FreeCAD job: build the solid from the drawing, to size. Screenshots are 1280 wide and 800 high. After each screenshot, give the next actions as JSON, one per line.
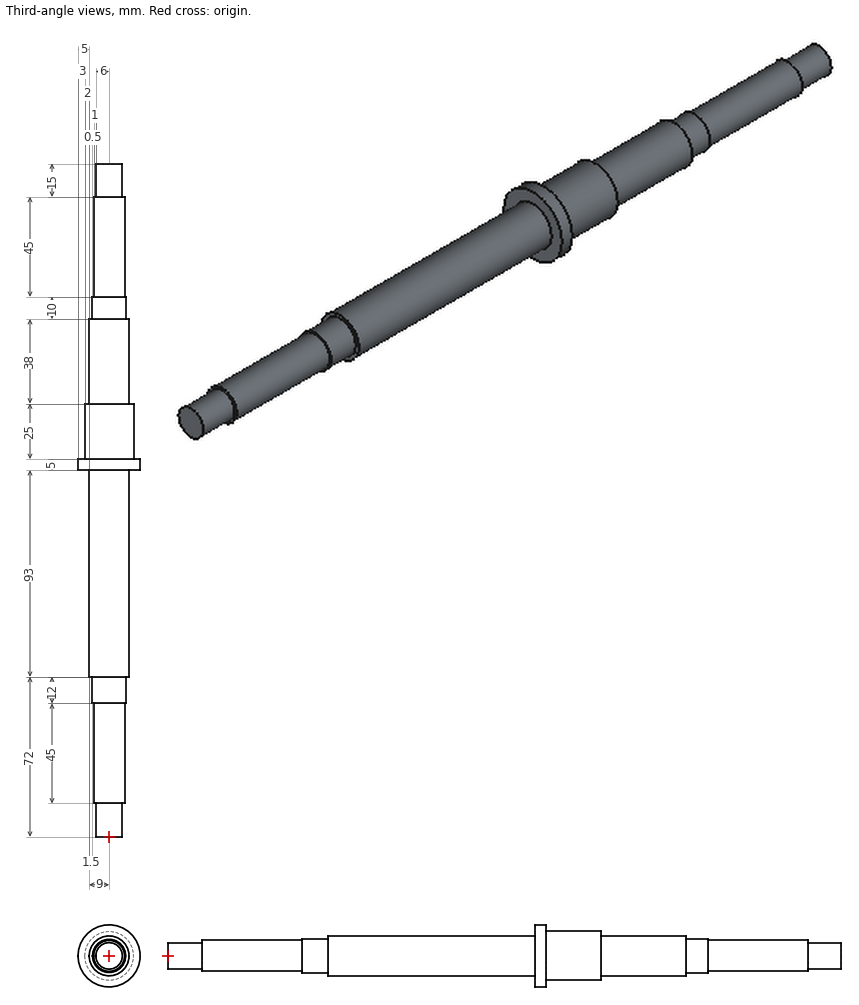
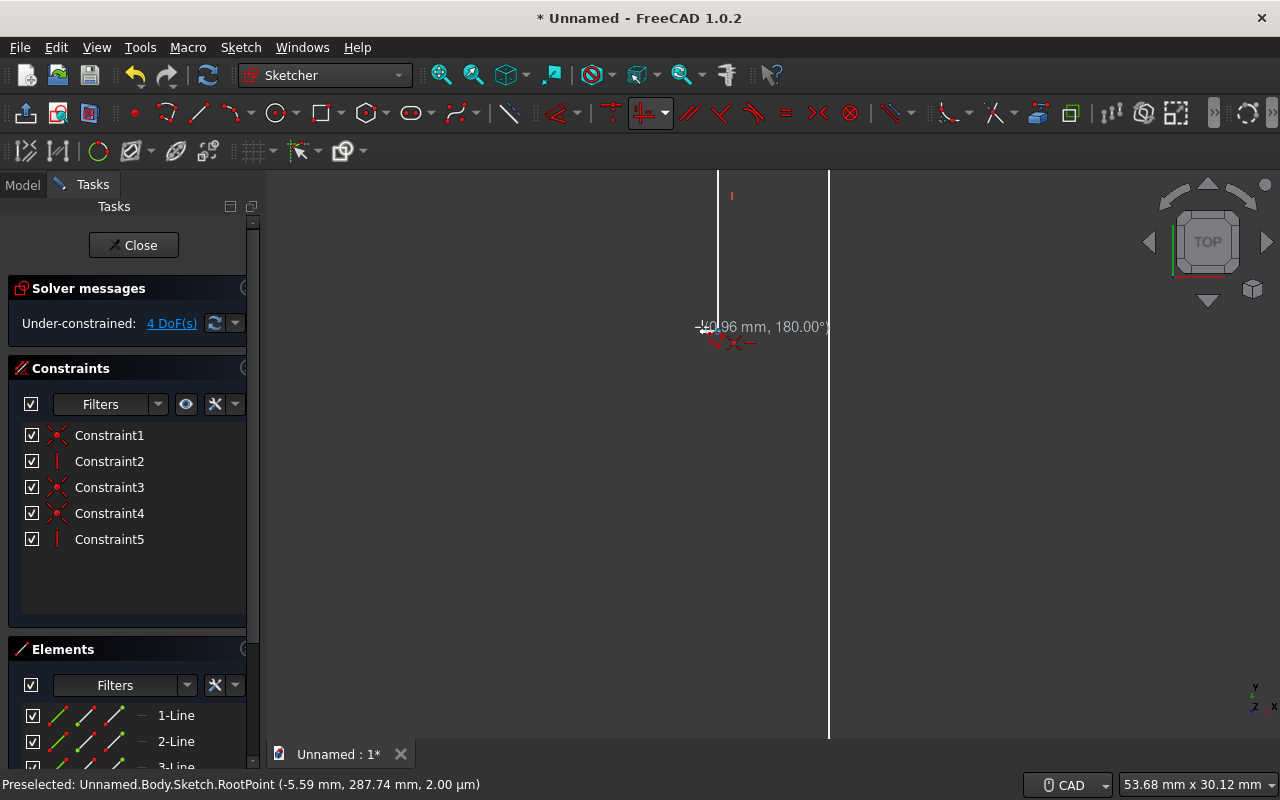
{"action": "left_click", "coordinate": [697, 326]}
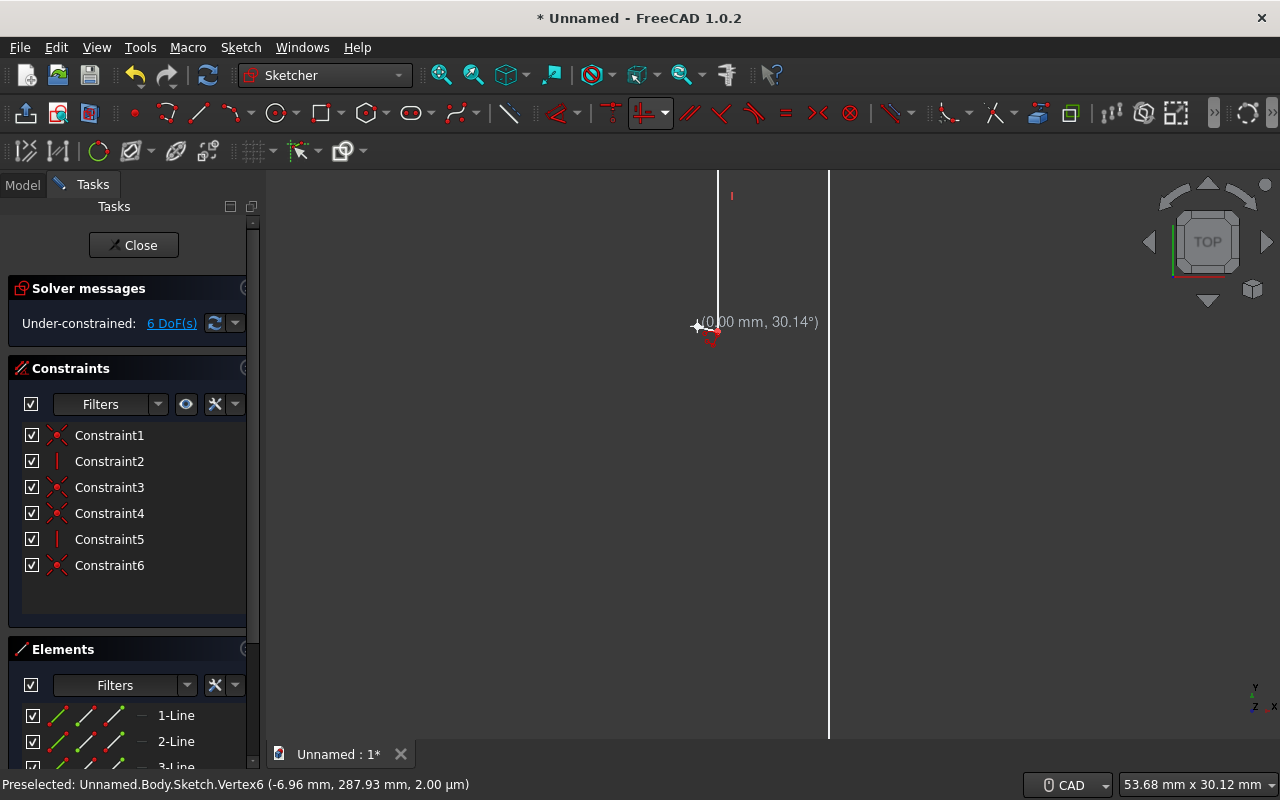
{"action": "scroll", "coordinate": [705, 296], "scroll_direction": "down", "scroll_amount": 14}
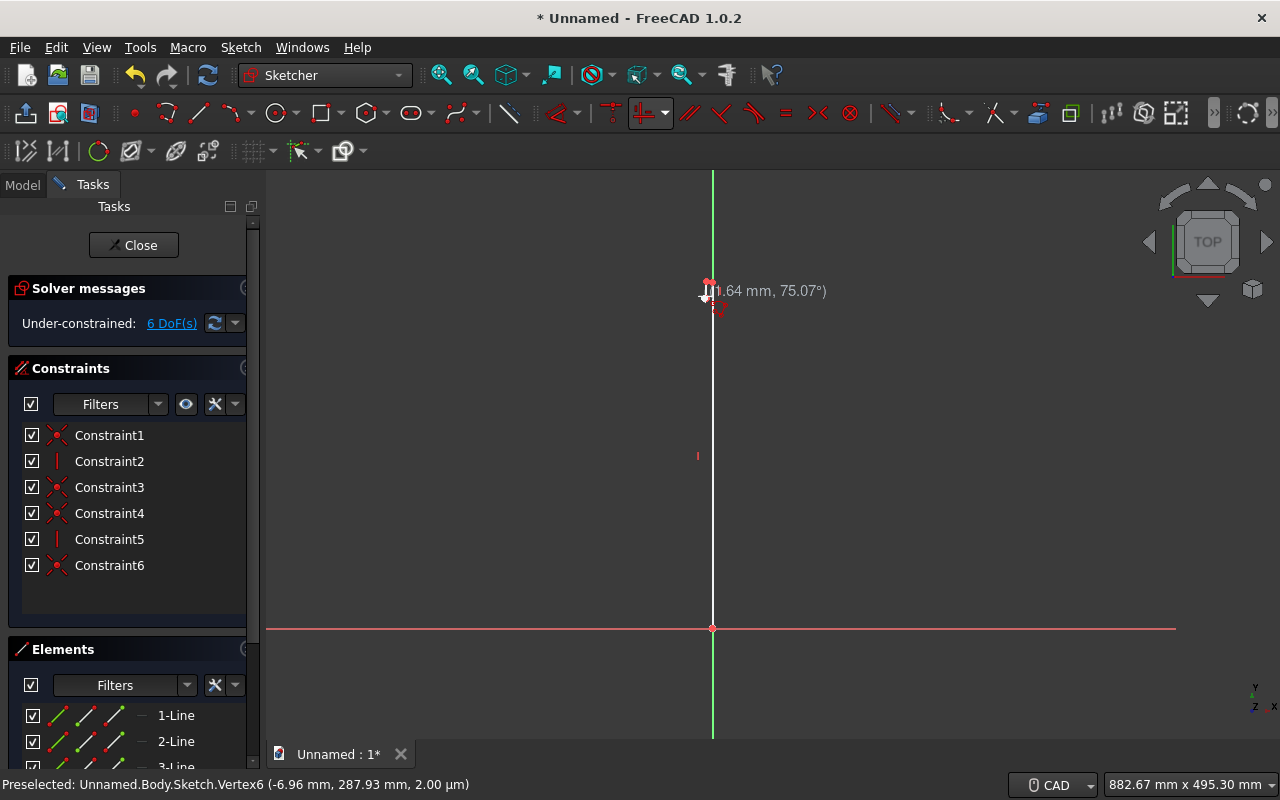
{"action": "scroll", "coordinate": [705, 350], "scroll_direction": "up", "scroll_amount": 4}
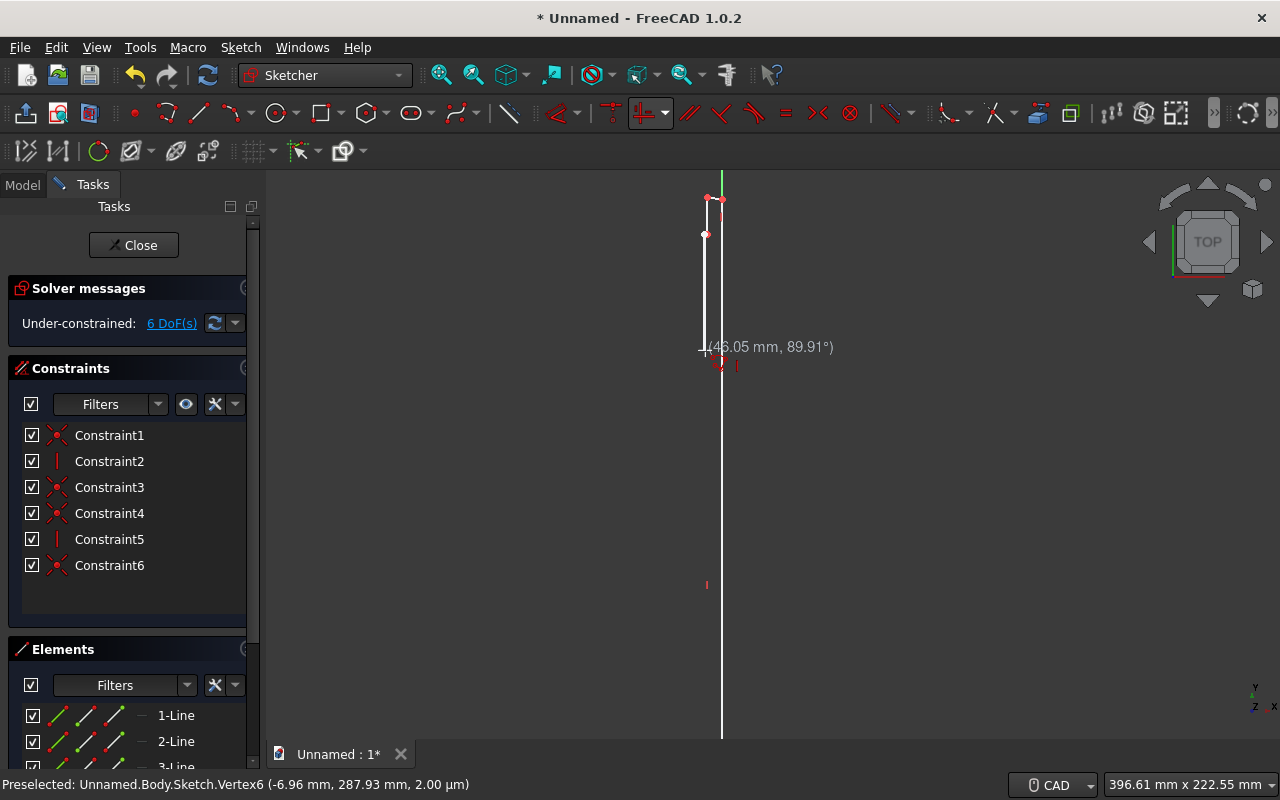
{"action": "left_click", "coordinate": [704, 349]}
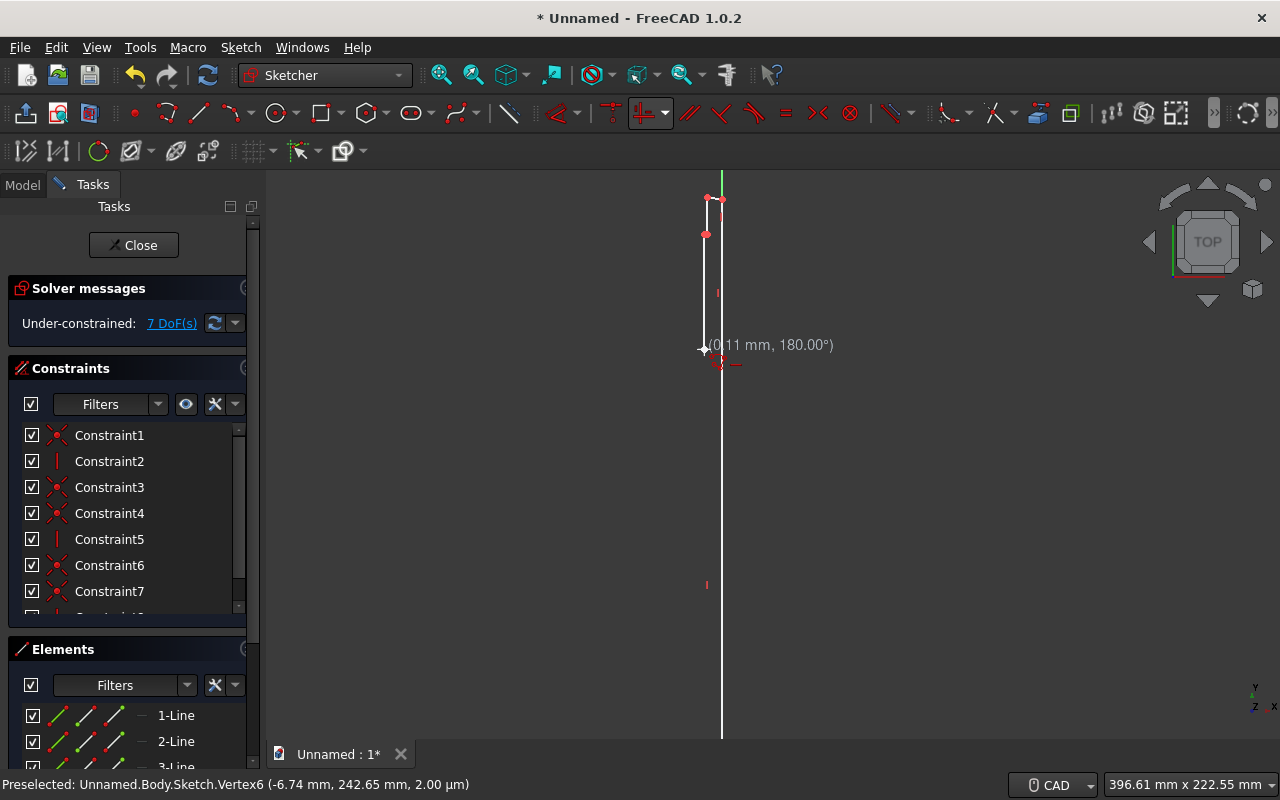
{"action": "scroll", "coordinate": [703, 349], "scroll_direction": "up", "scroll_amount": 13}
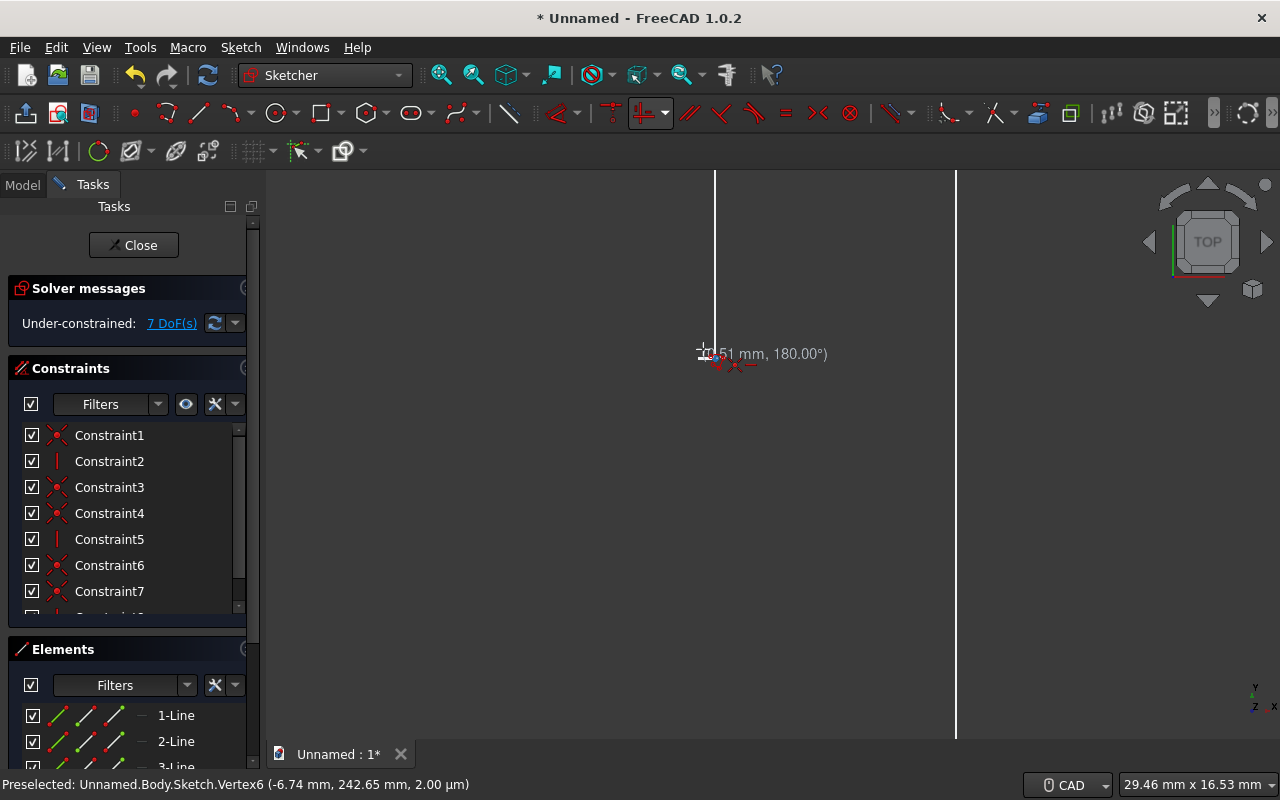
{"action": "left_click", "coordinate": [698, 345]}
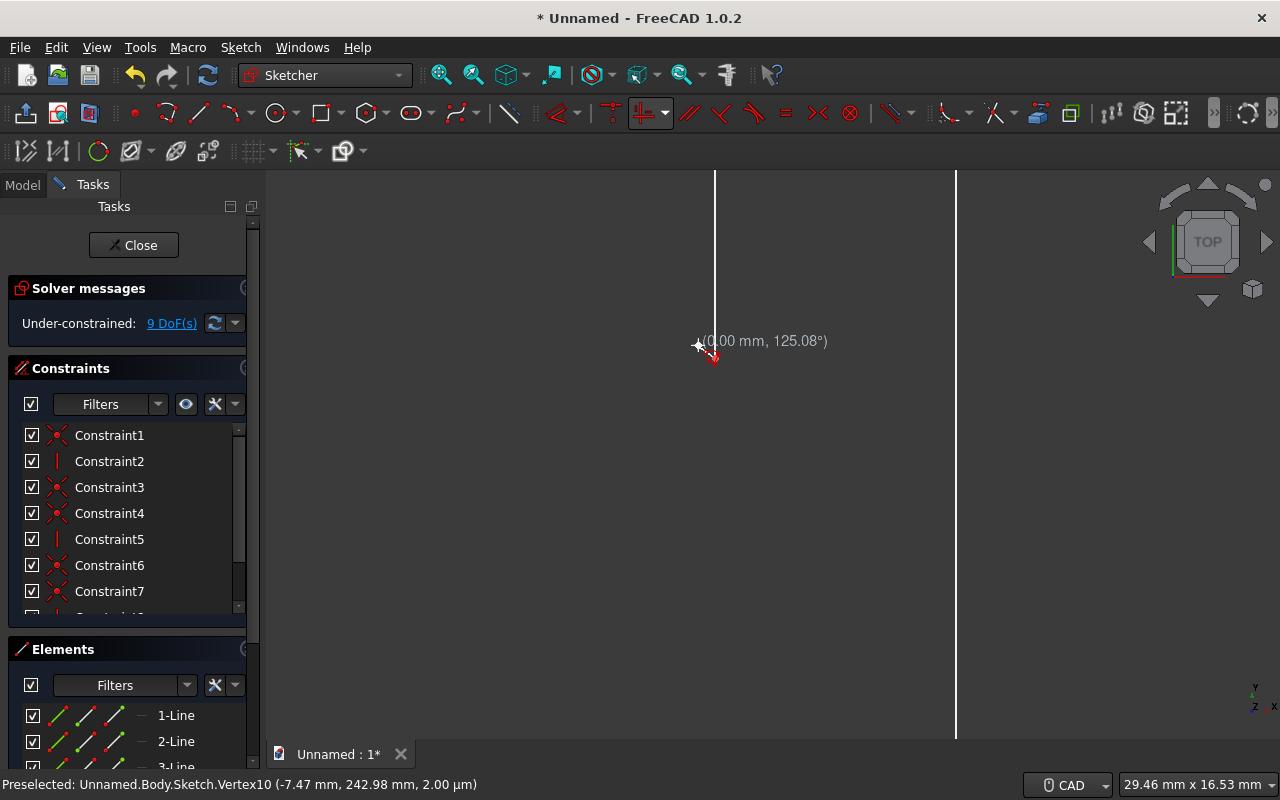
{"action": "scroll", "coordinate": [704, 325], "scroll_direction": "down", "scroll_amount": 16}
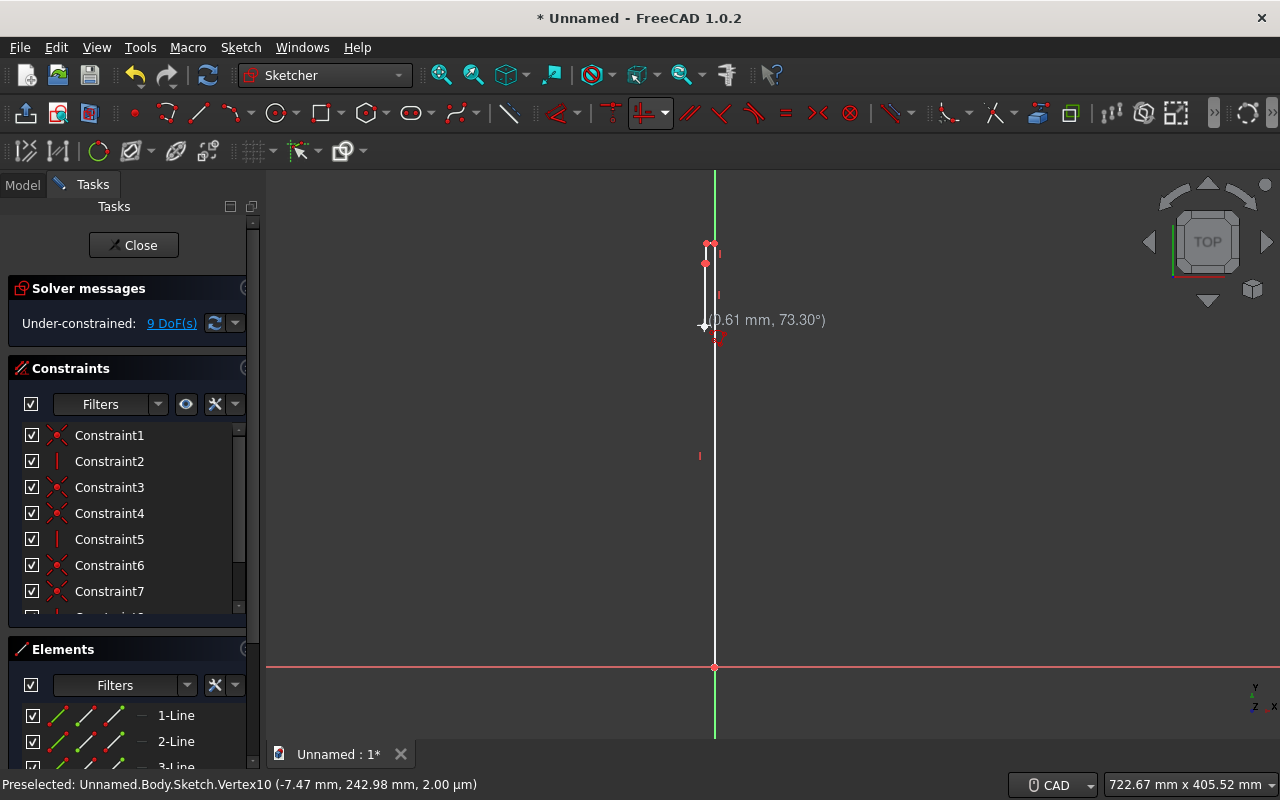
{"action": "scroll", "coordinate": [704, 340], "scroll_direction": "up", "scroll_amount": 3}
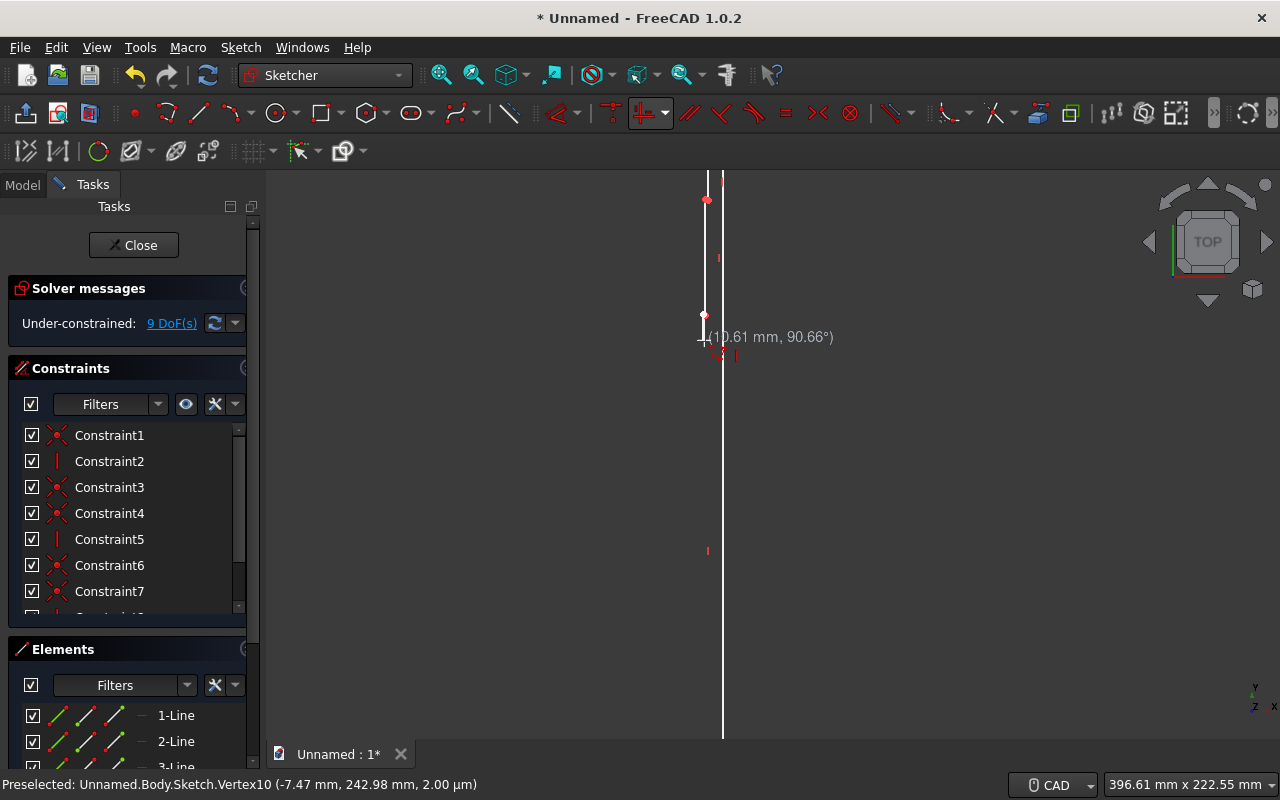
{"action": "left_click", "coordinate": [704, 340]}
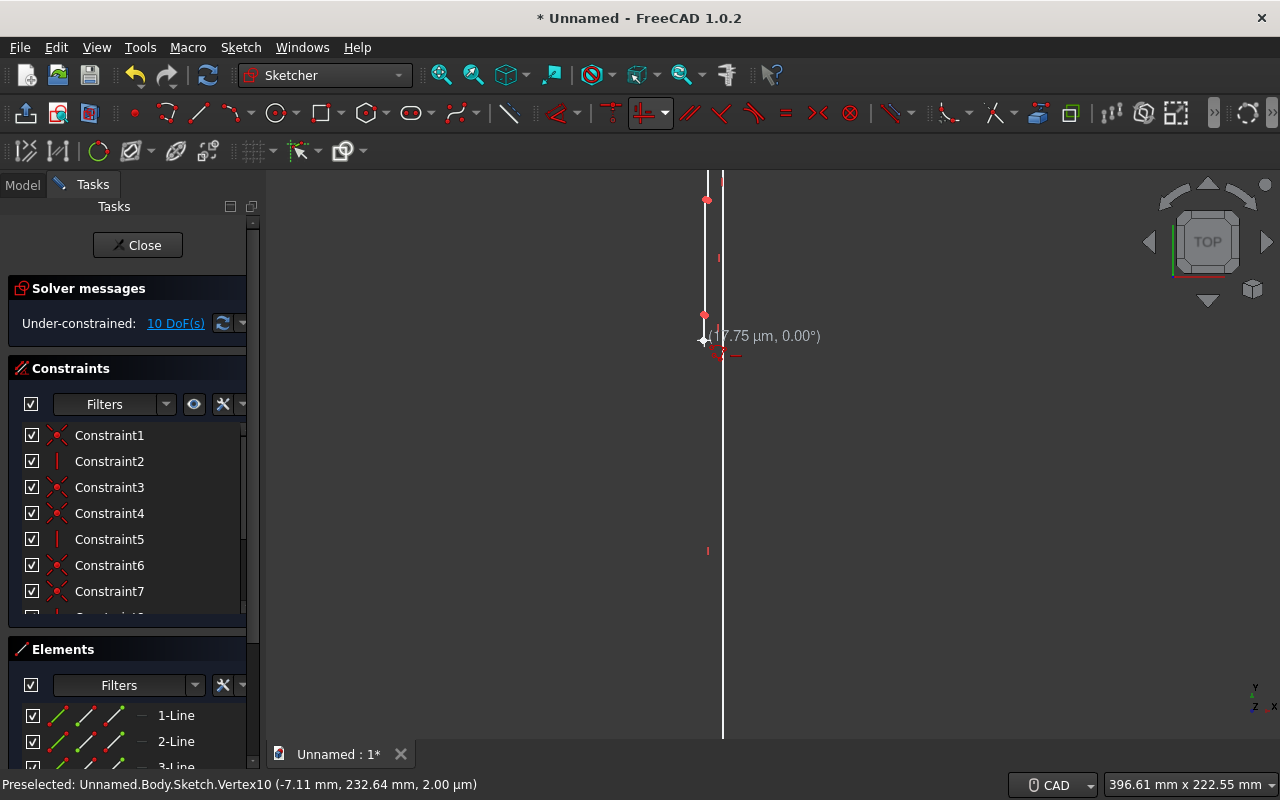
{"action": "scroll", "coordinate": [700, 340], "scroll_direction": "up", "scroll_amount": 8}